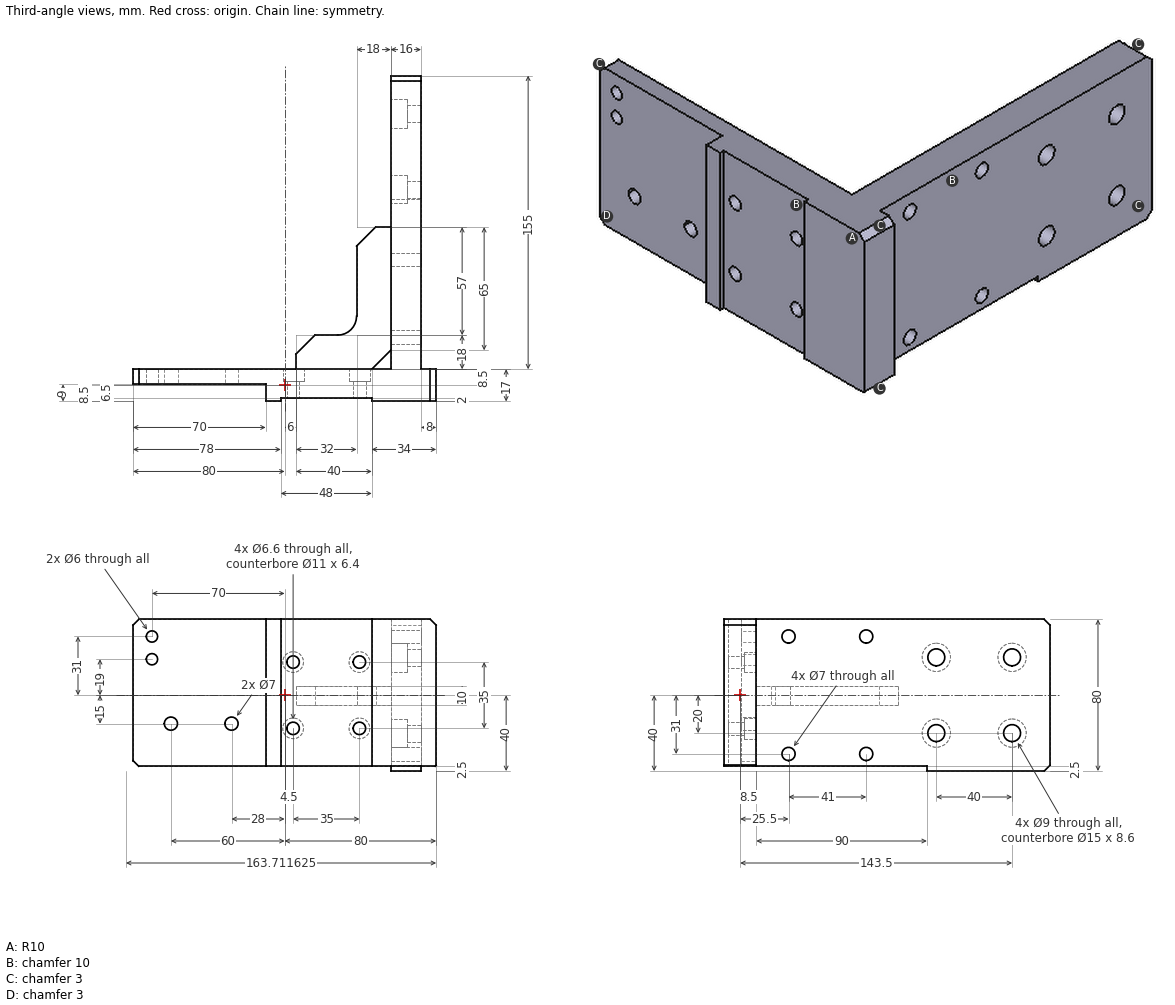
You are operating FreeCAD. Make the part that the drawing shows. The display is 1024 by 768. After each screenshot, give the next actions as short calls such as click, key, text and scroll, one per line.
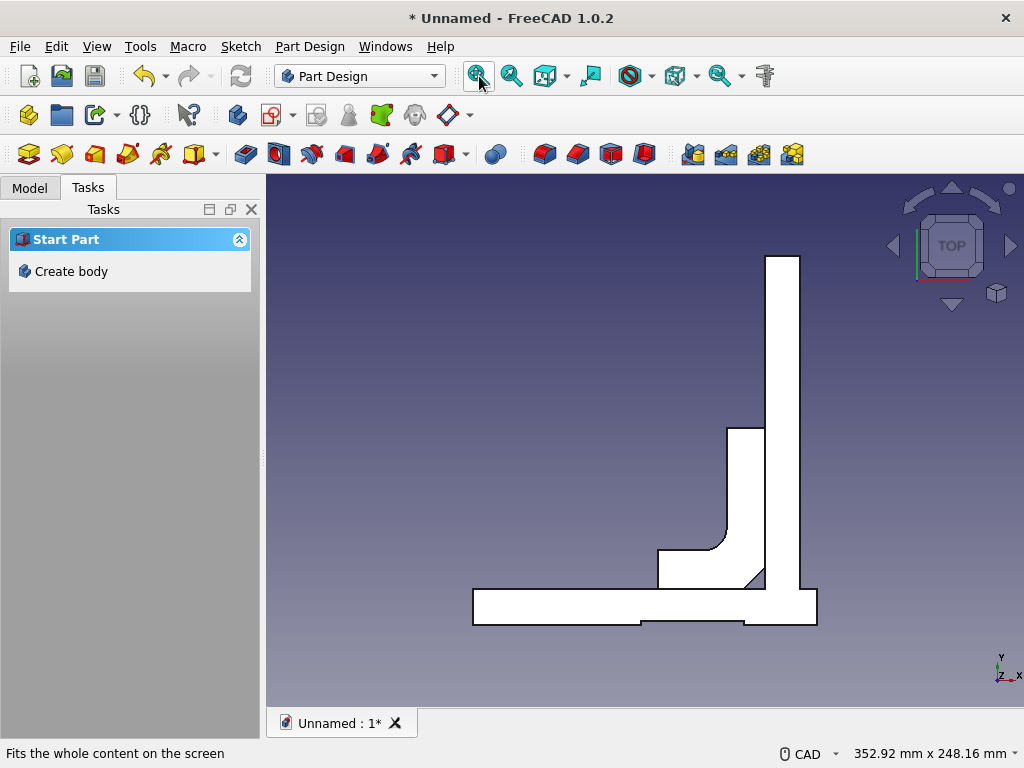
key(1)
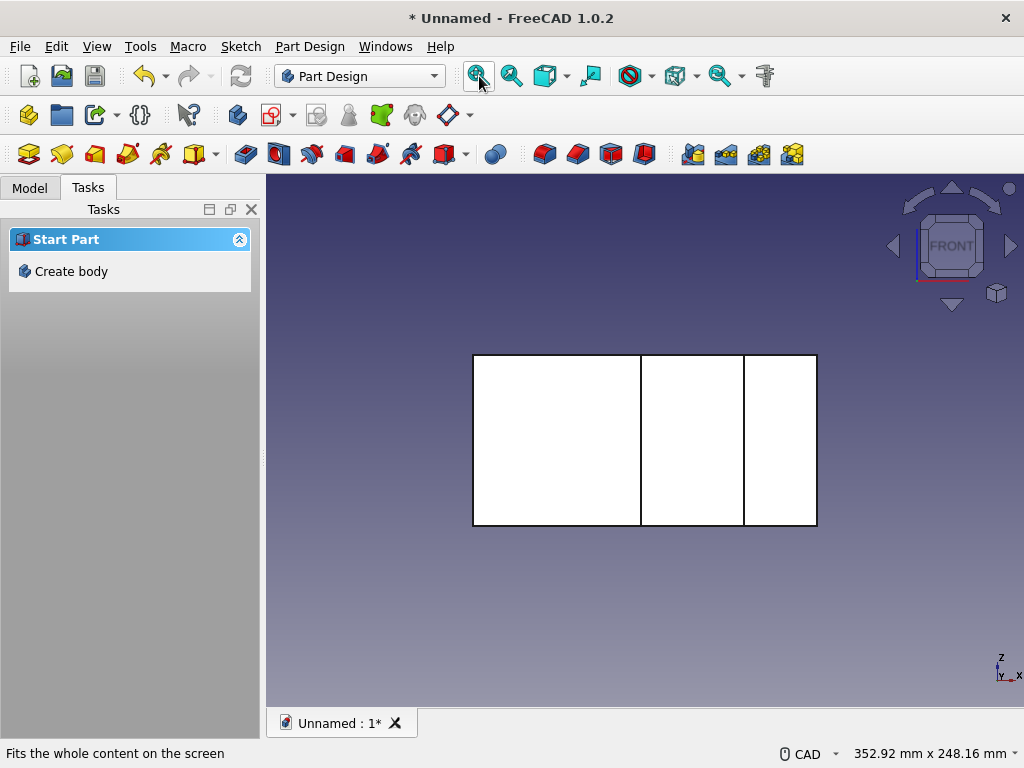
scroll(658, 440, up, 4)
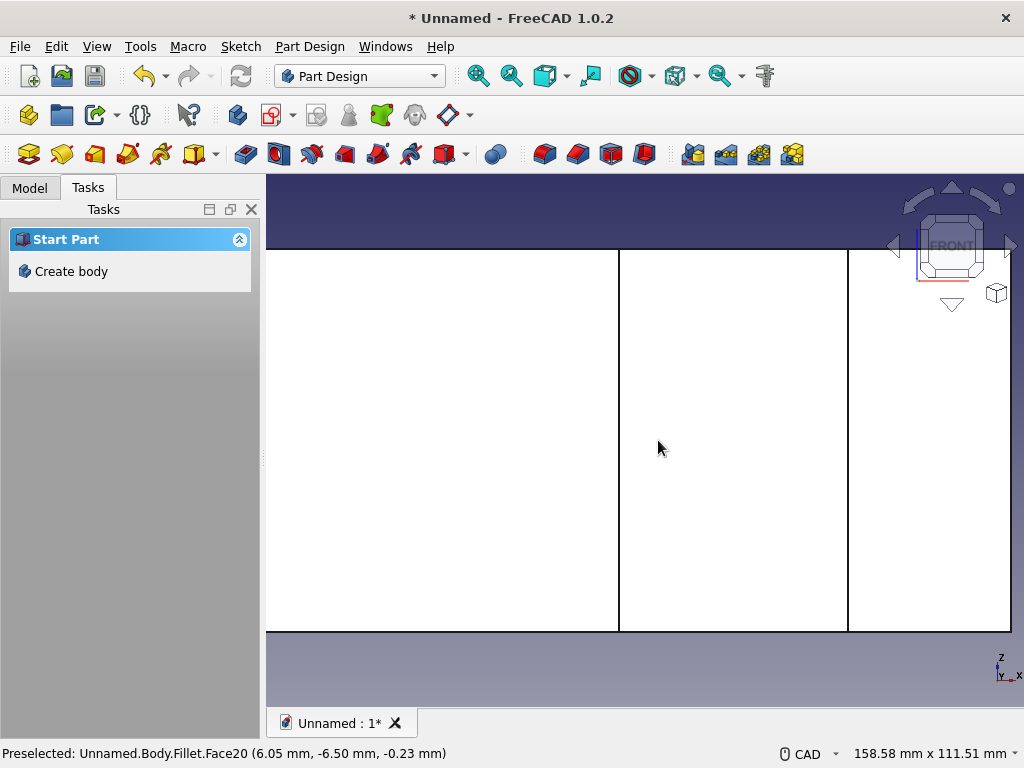
click(479, 76)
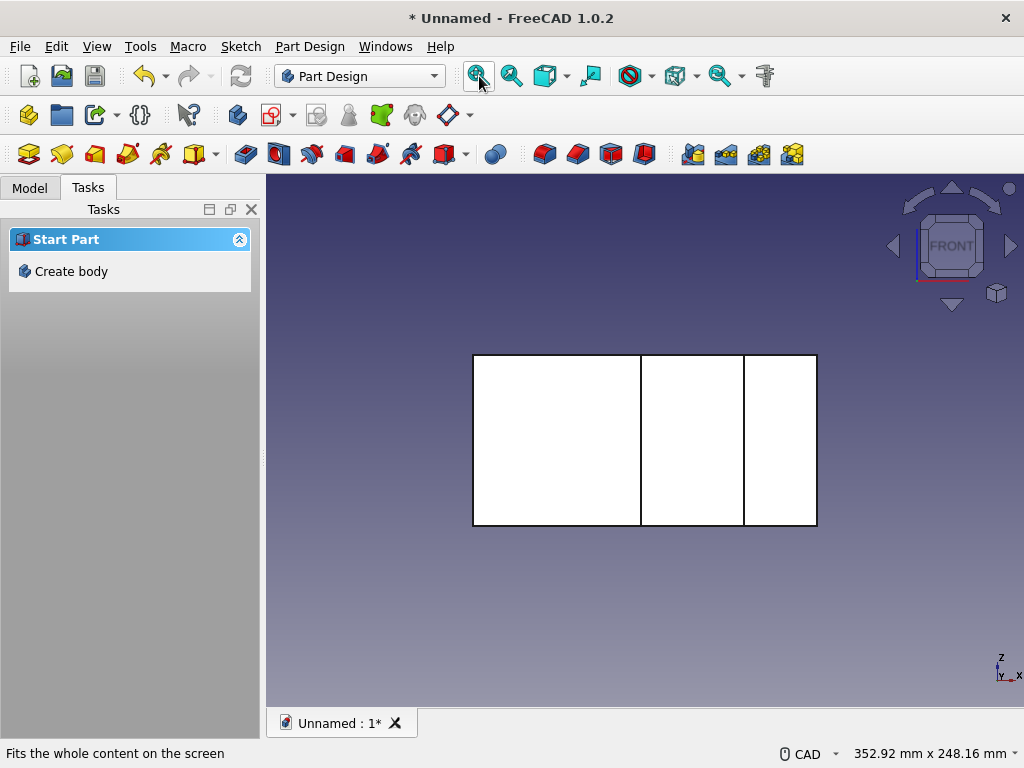
key(3)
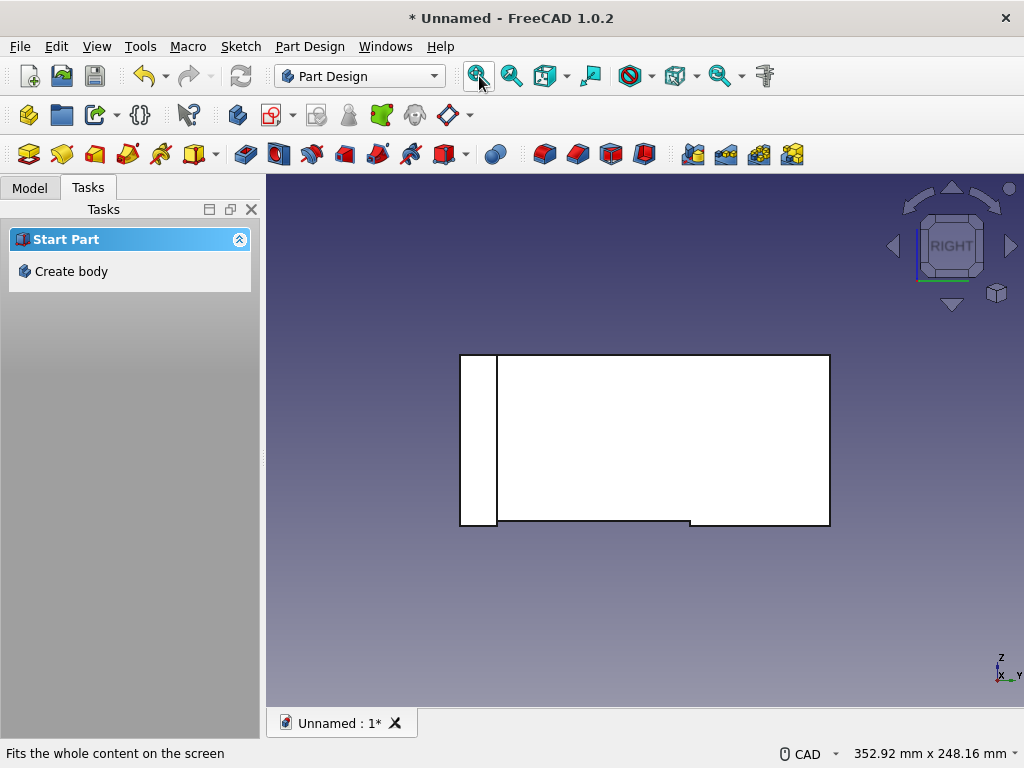
scroll(535, 439, up, 4)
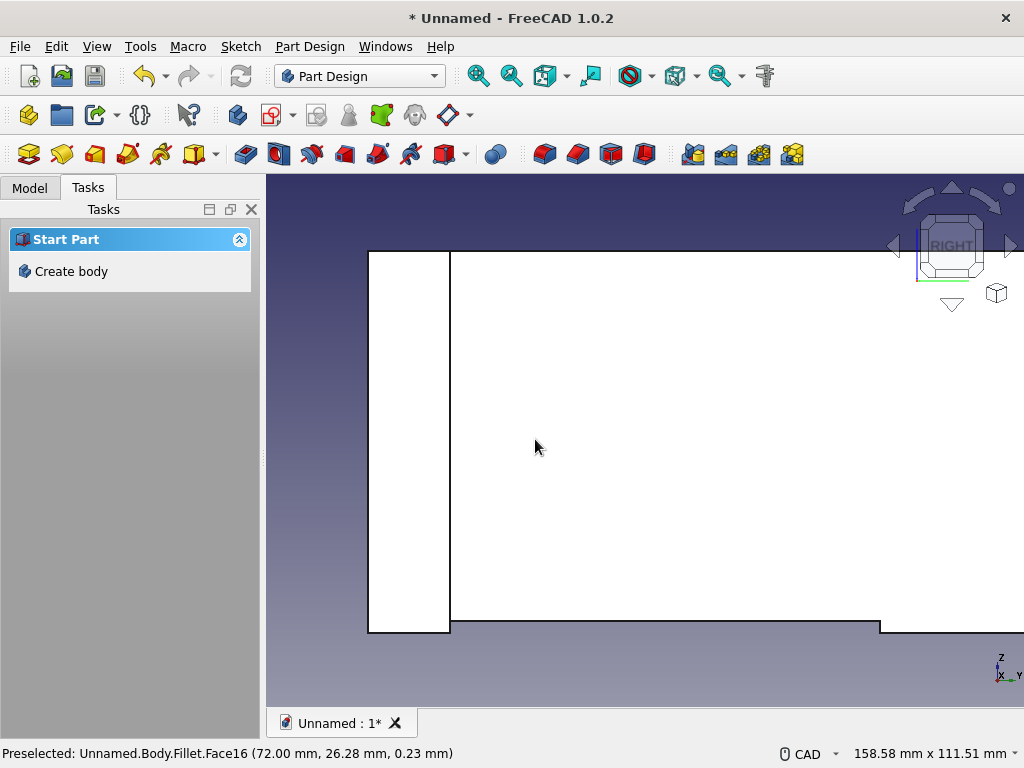
click(479, 76)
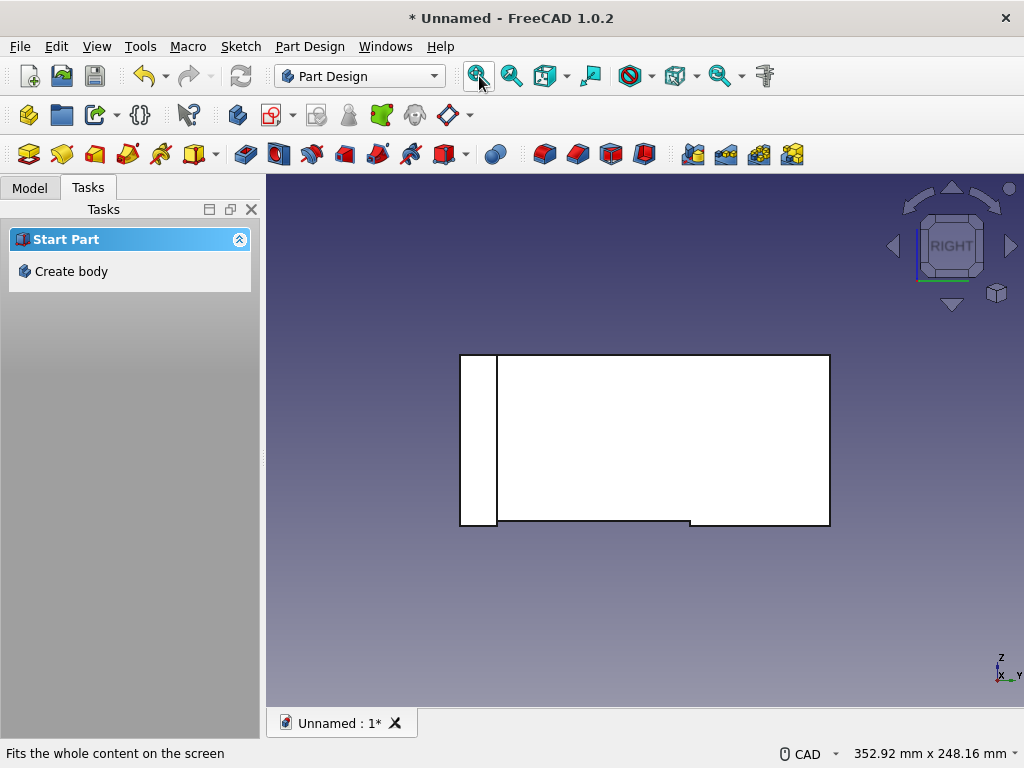
key(5)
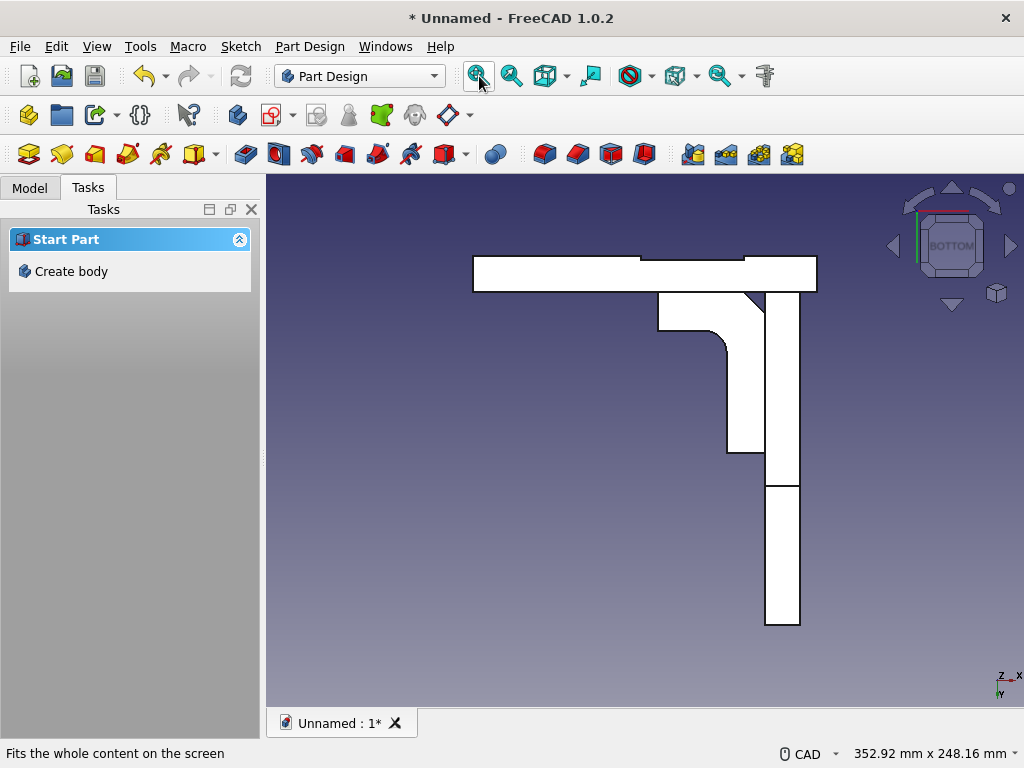
scroll(658, 330, up, 4)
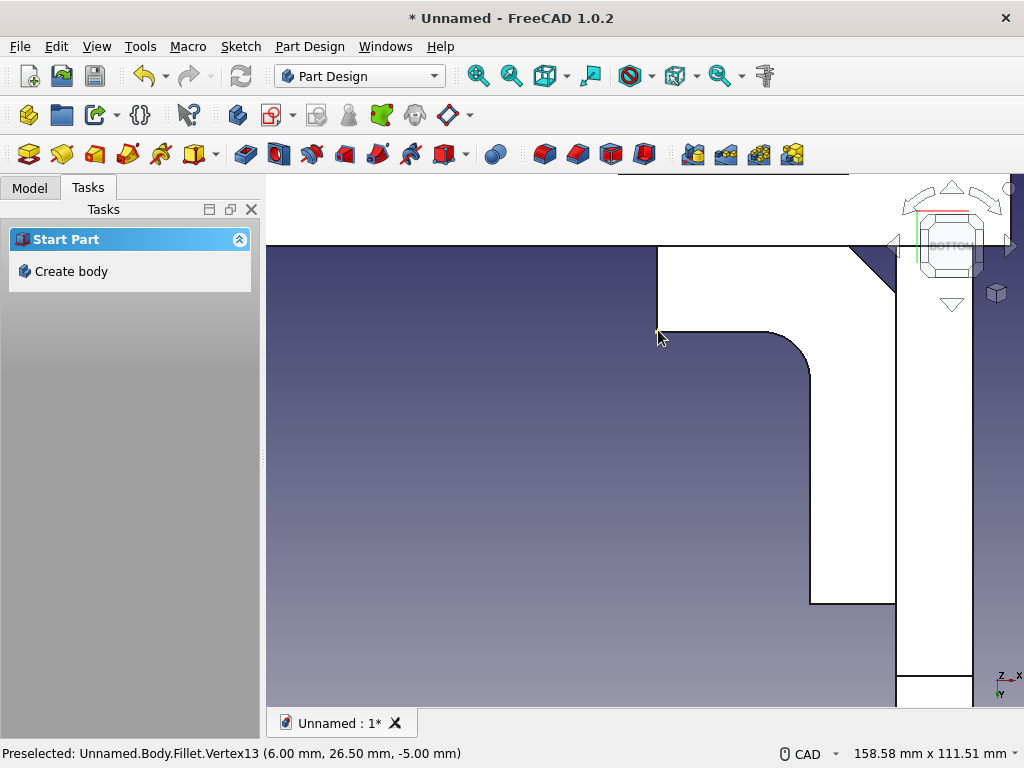
key(v)
key(f)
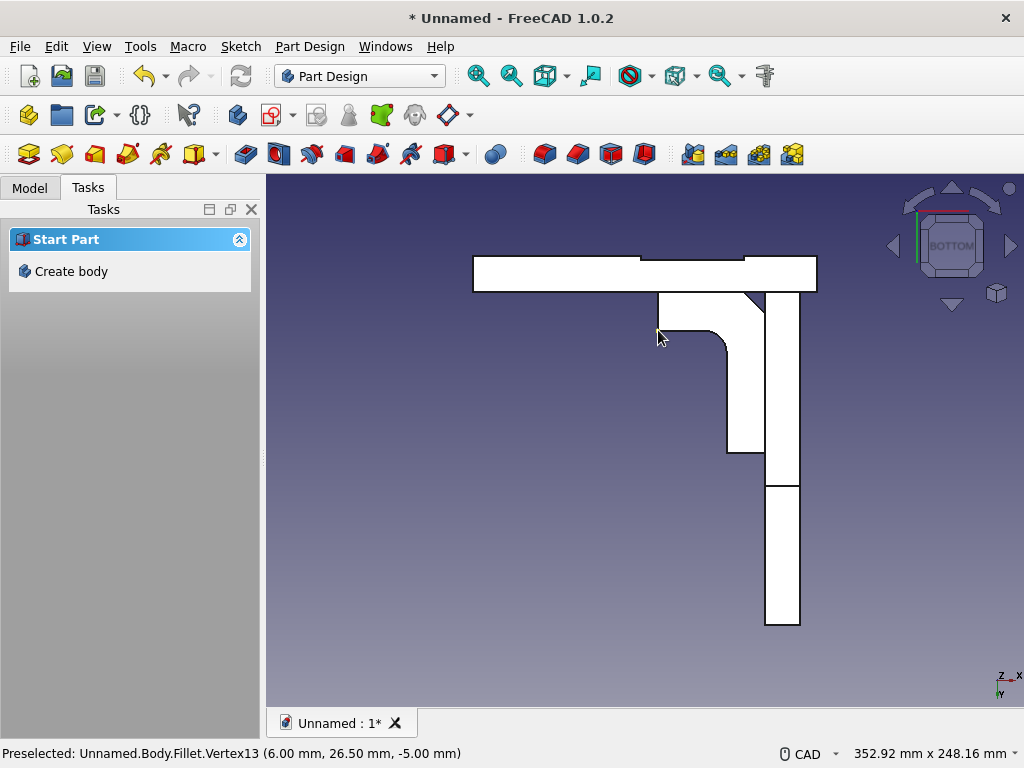
key(4)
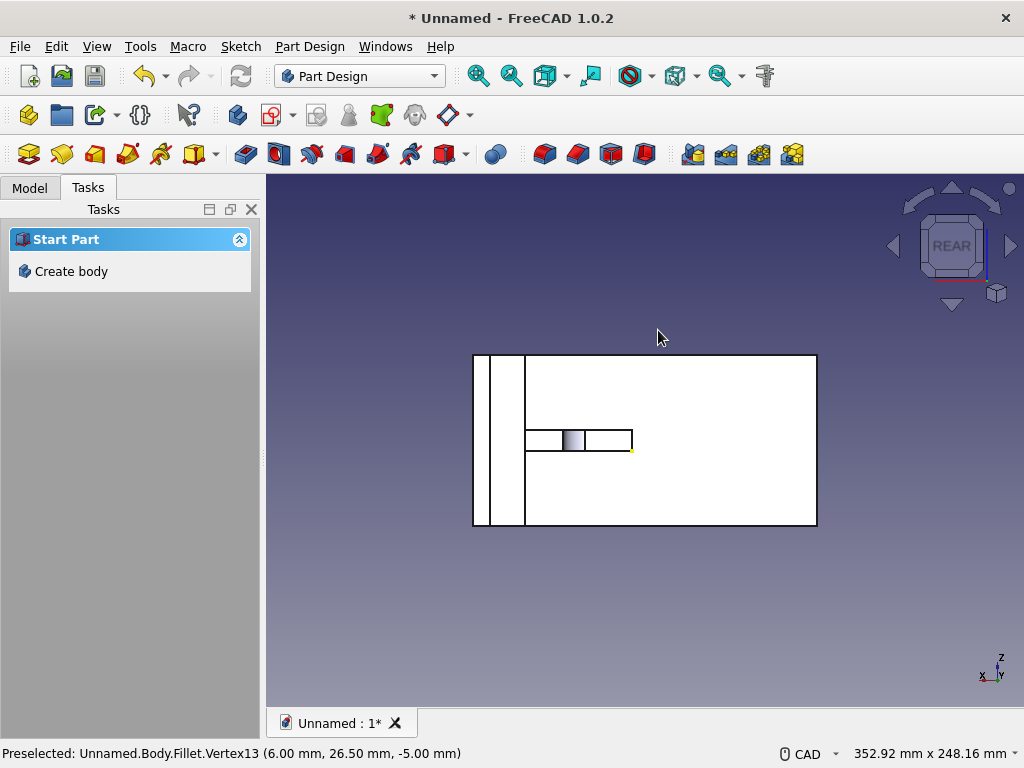
click(632, 440)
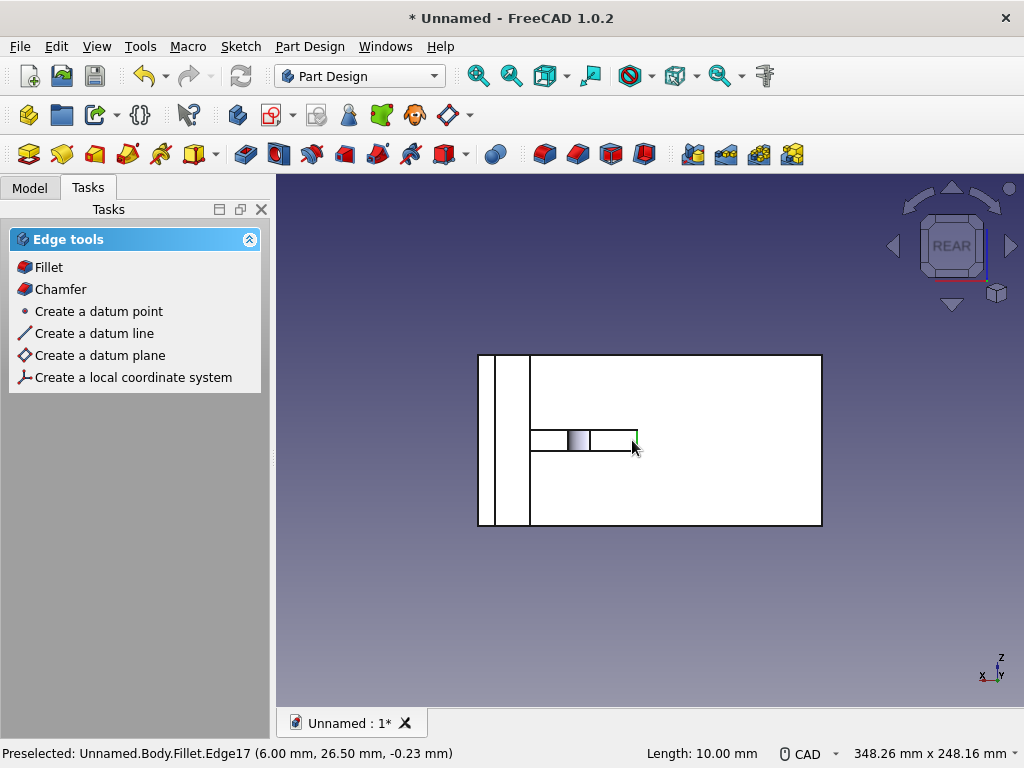
click(568, 440, ctrl)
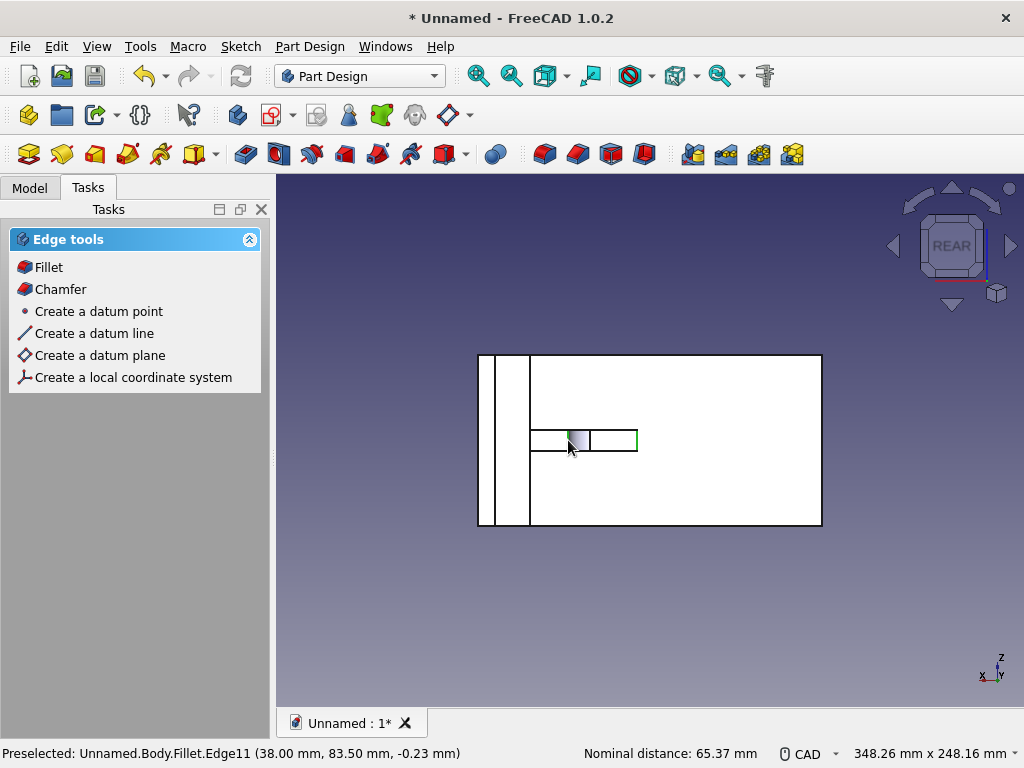
click(578, 154)